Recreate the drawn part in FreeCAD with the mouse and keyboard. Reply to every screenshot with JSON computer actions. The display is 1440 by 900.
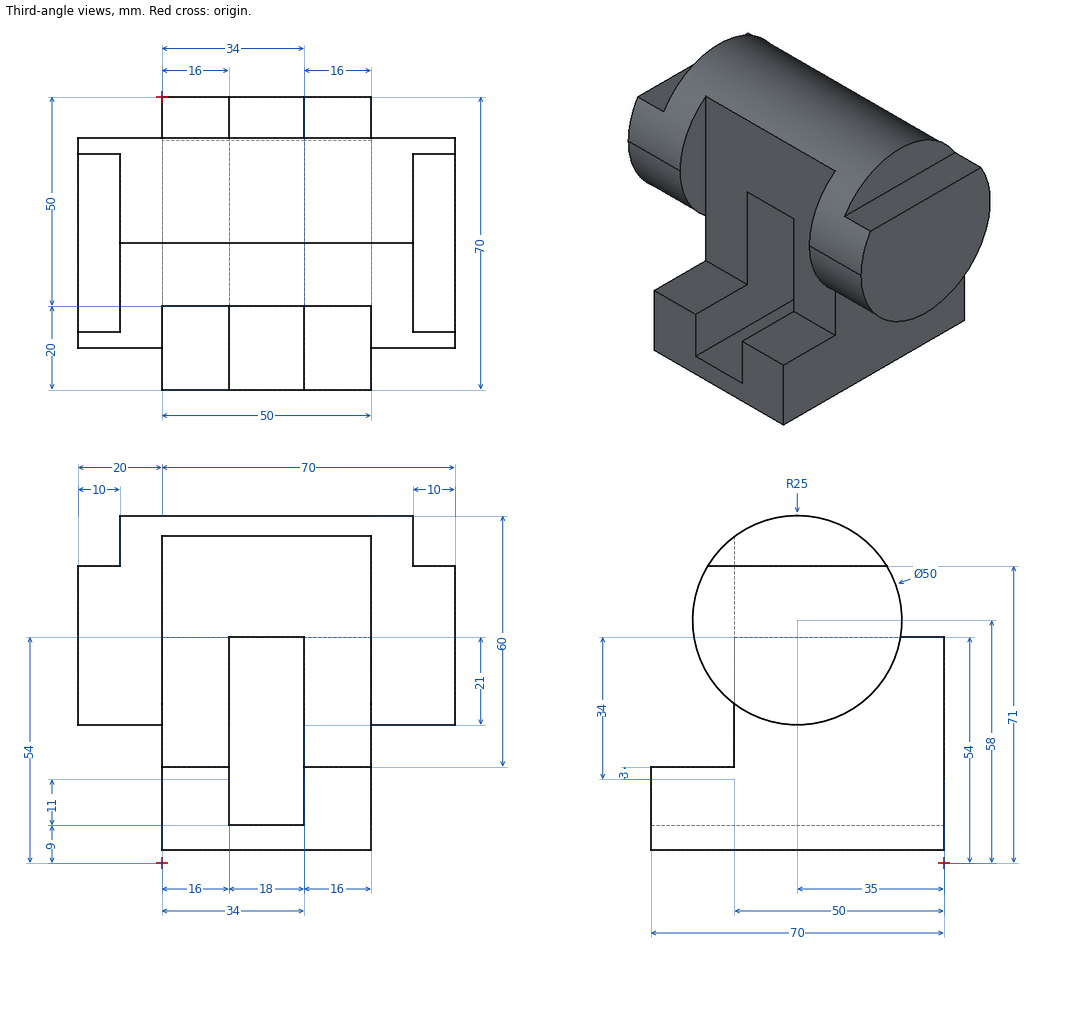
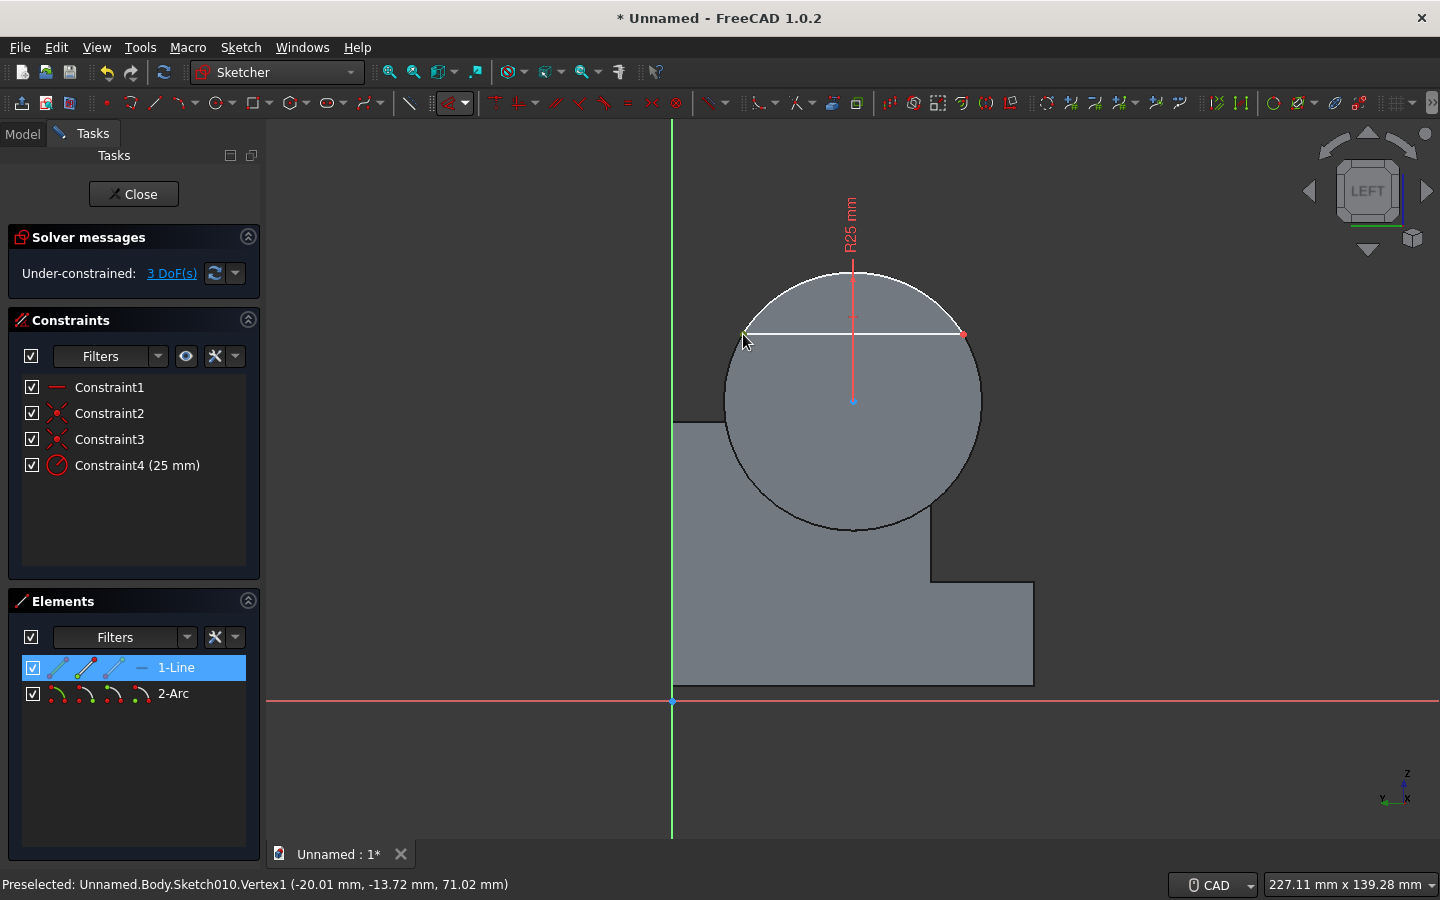
{"action": "key", "text": "i"}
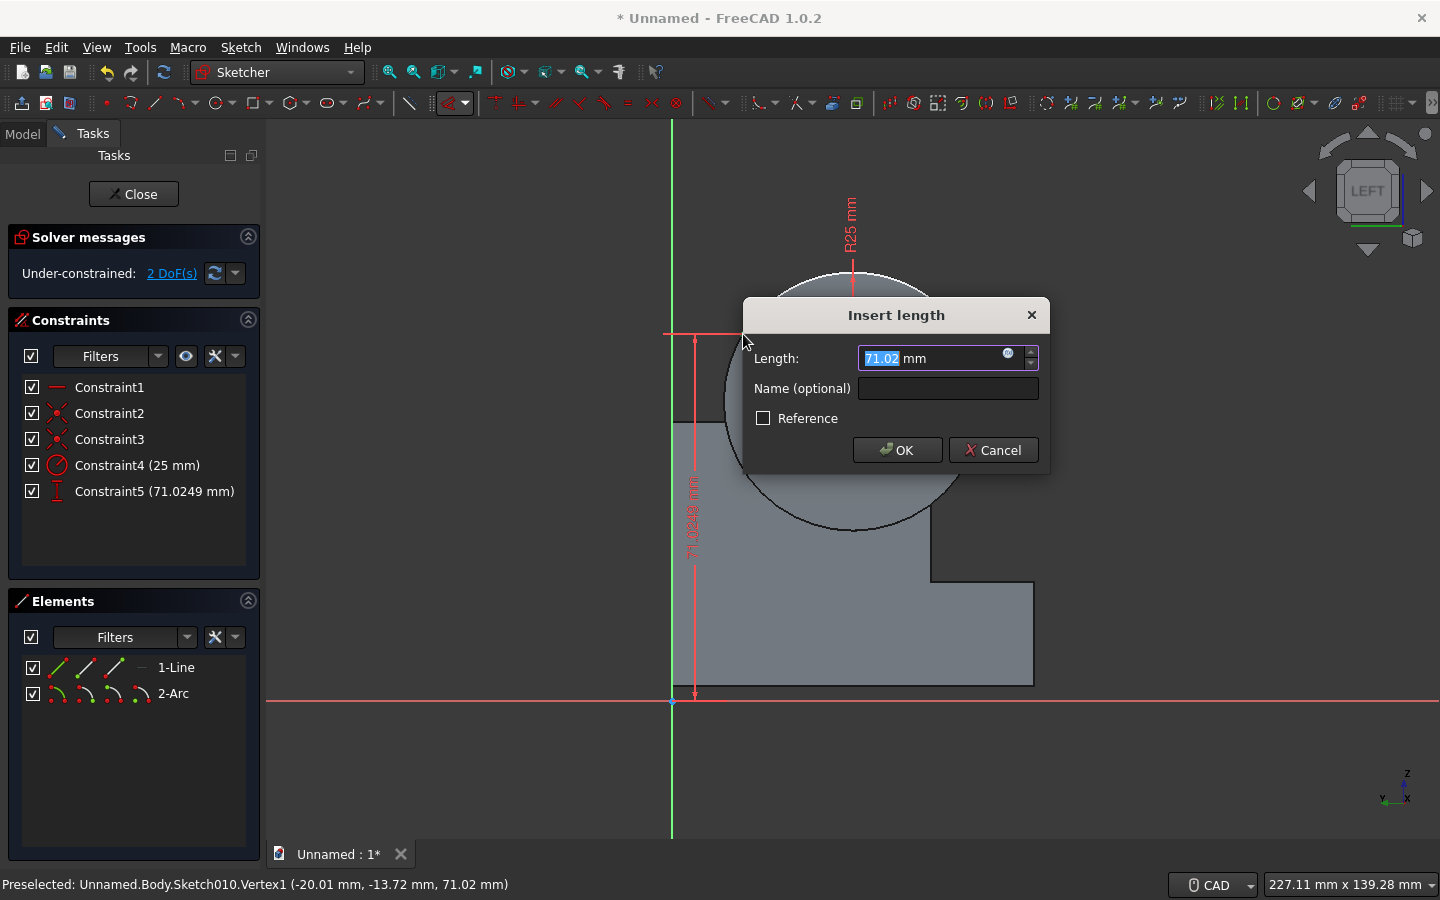
{"action": "type", "text": "71"}
{"action": "key", "text": "Return"}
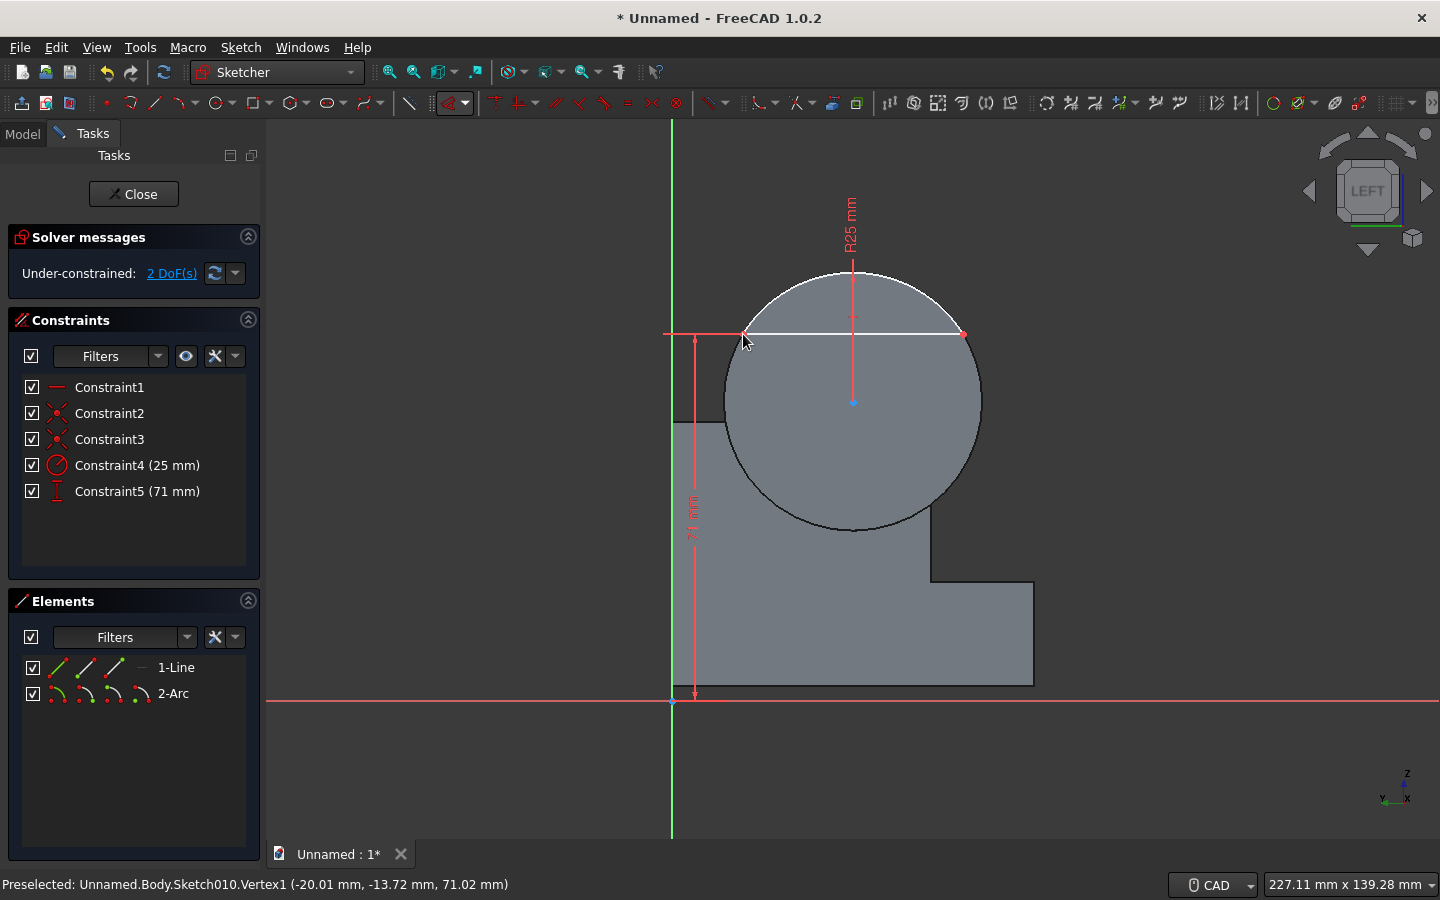
{"action": "left_click", "coordinate": [853, 402]}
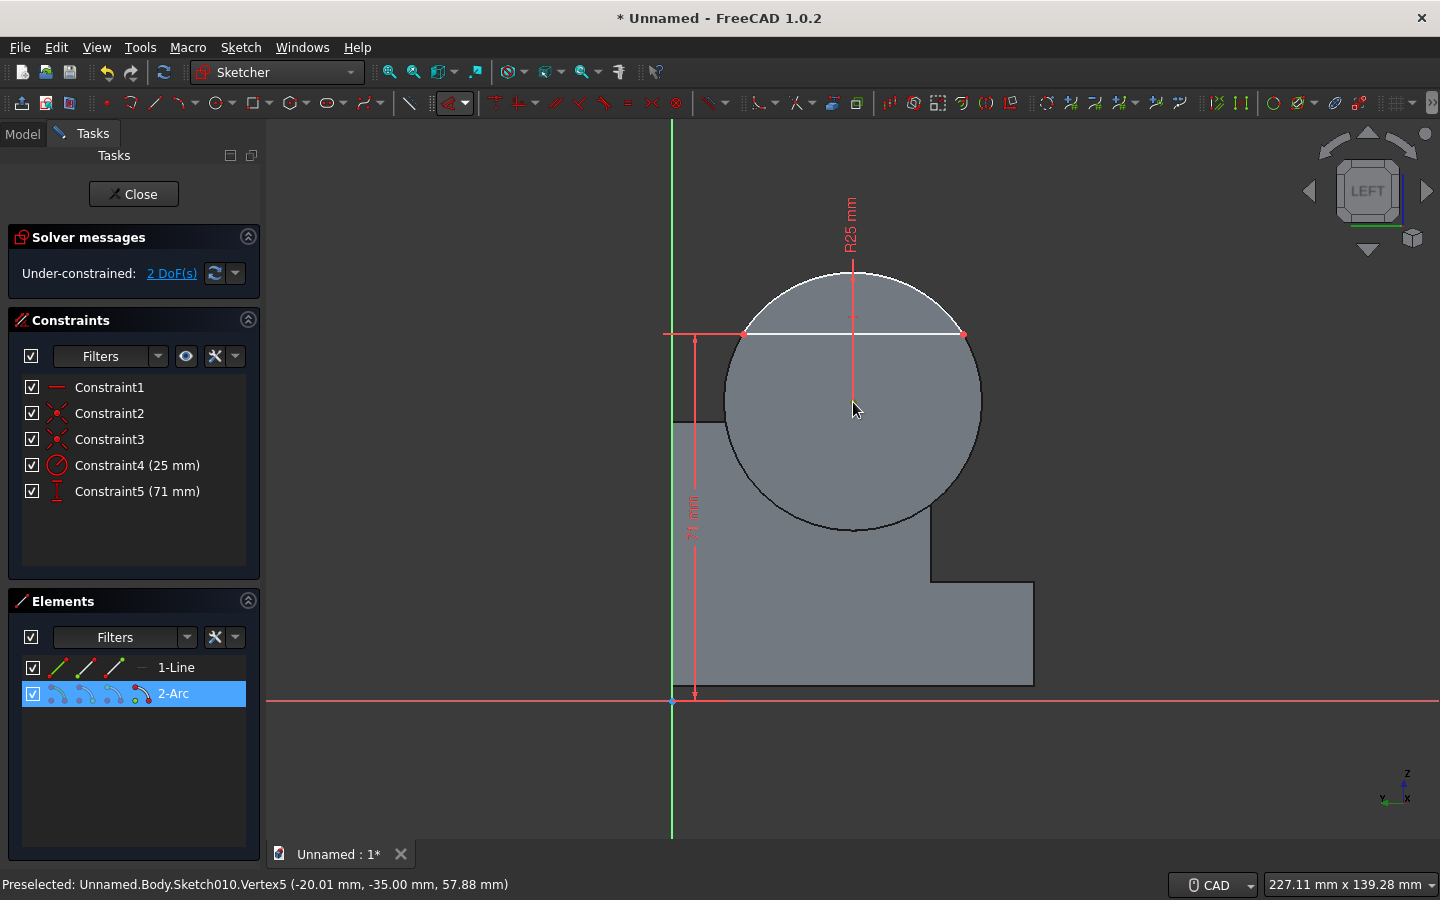
{"action": "key", "text": "l"}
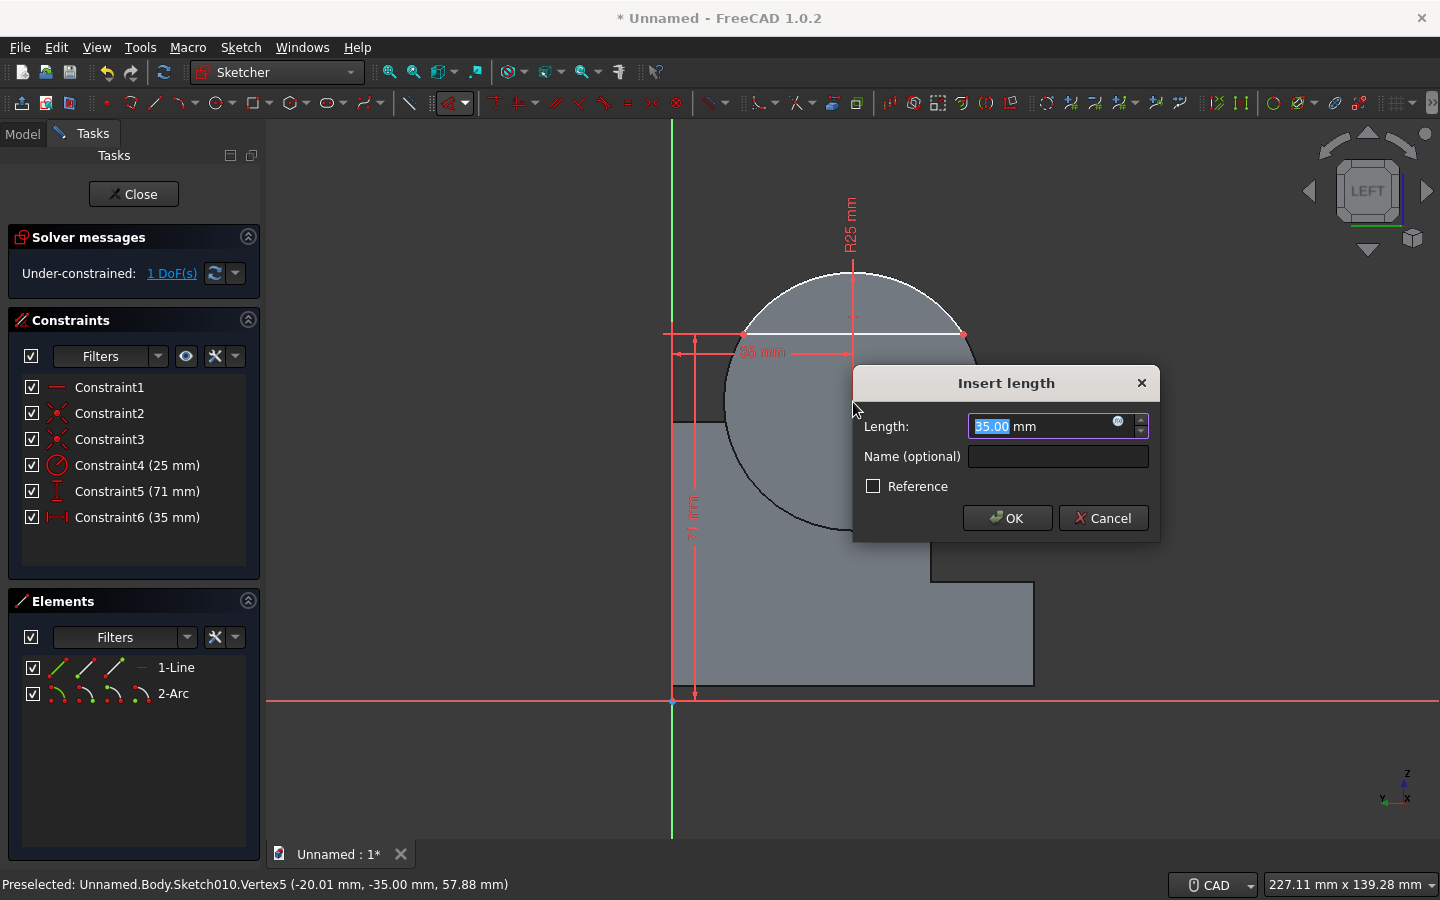
{"action": "type", "text": "35"}
{"action": "key", "text": "Return"}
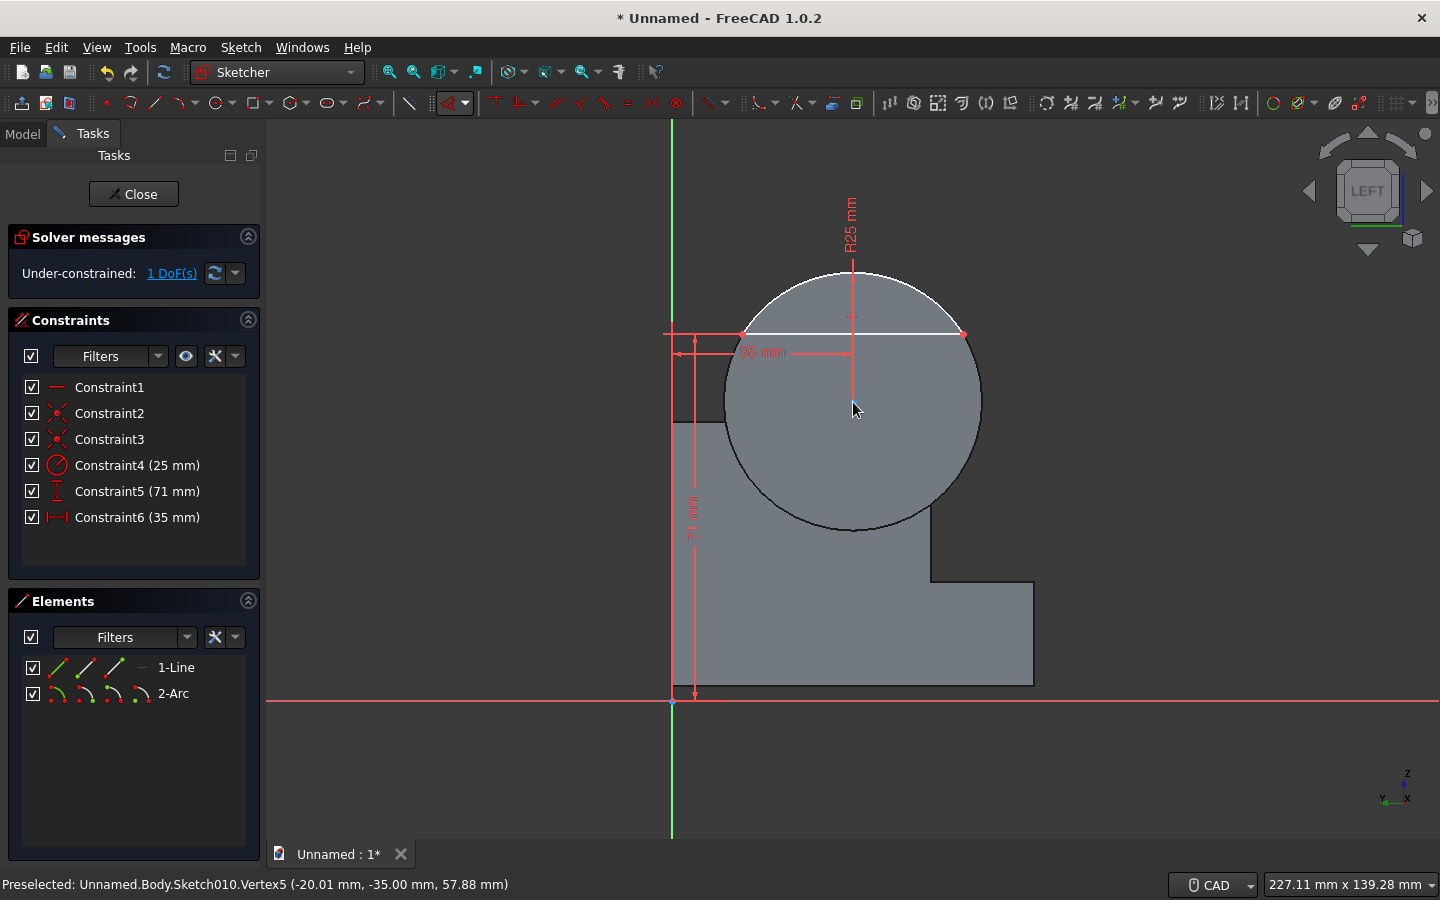
{"action": "left_click", "coordinate": [853, 402]}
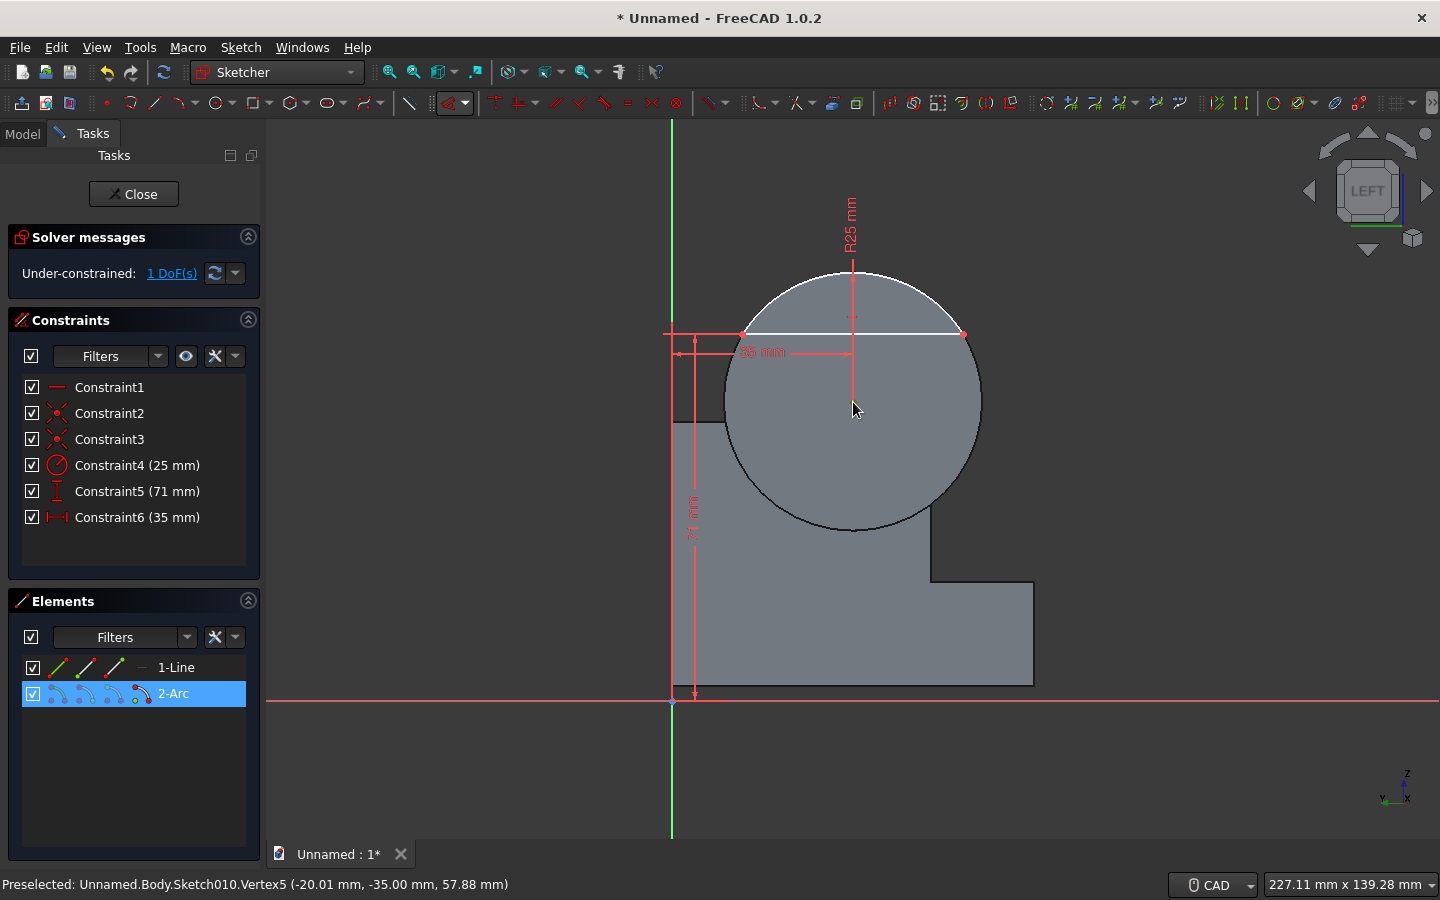
{"action": "key", "text": "i"}